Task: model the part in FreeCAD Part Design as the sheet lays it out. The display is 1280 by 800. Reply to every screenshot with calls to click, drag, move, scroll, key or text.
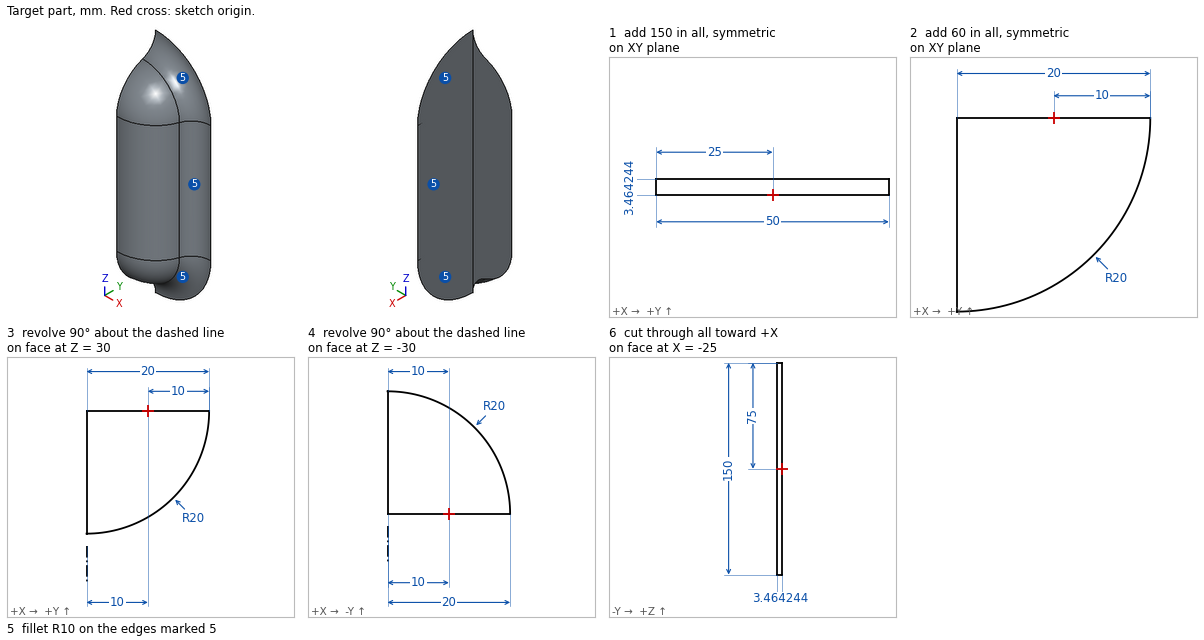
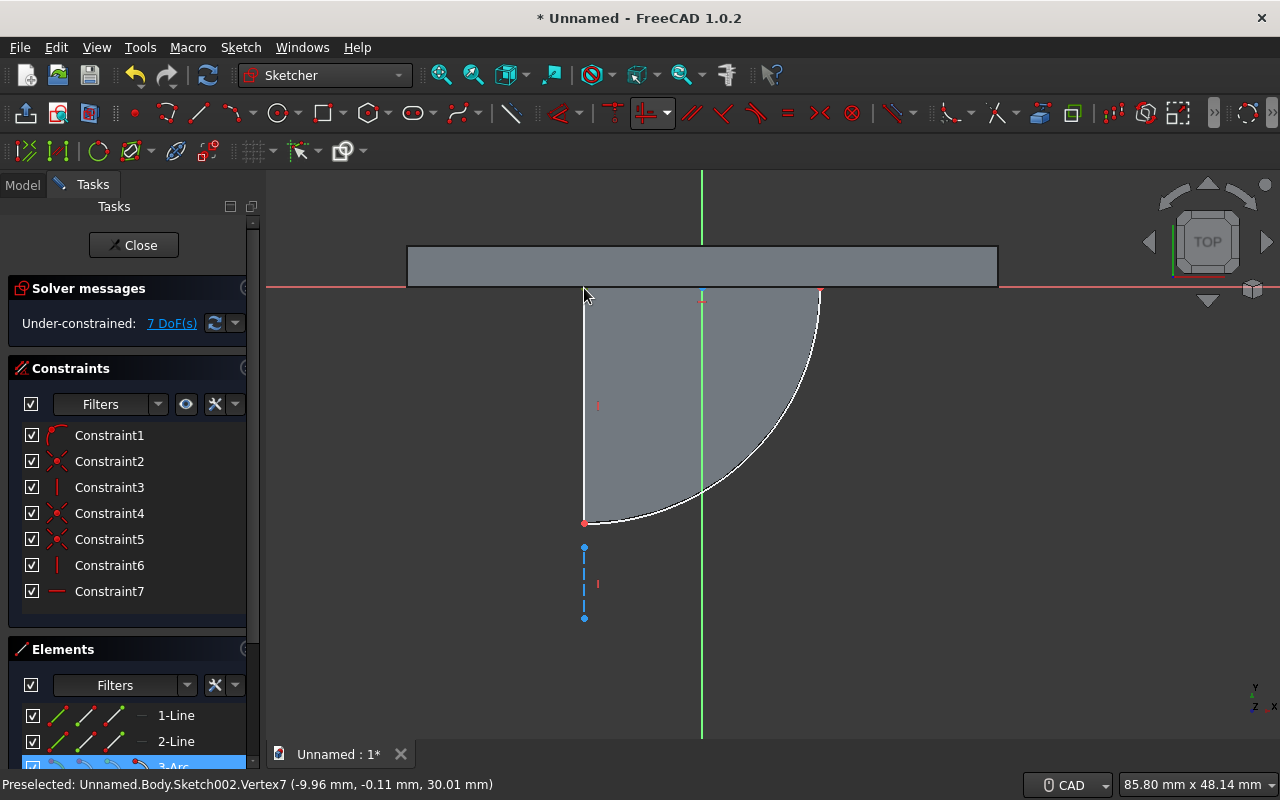
click(353, 287)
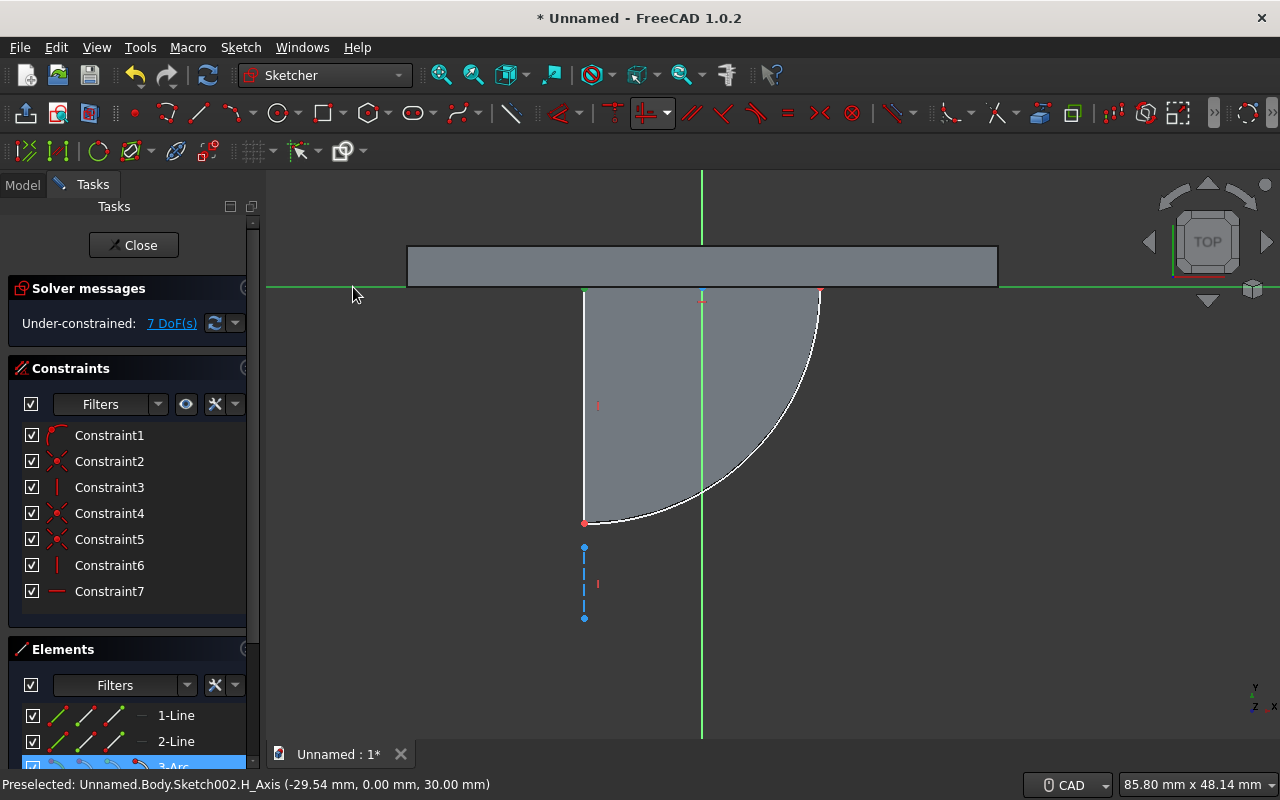
click(614, 114)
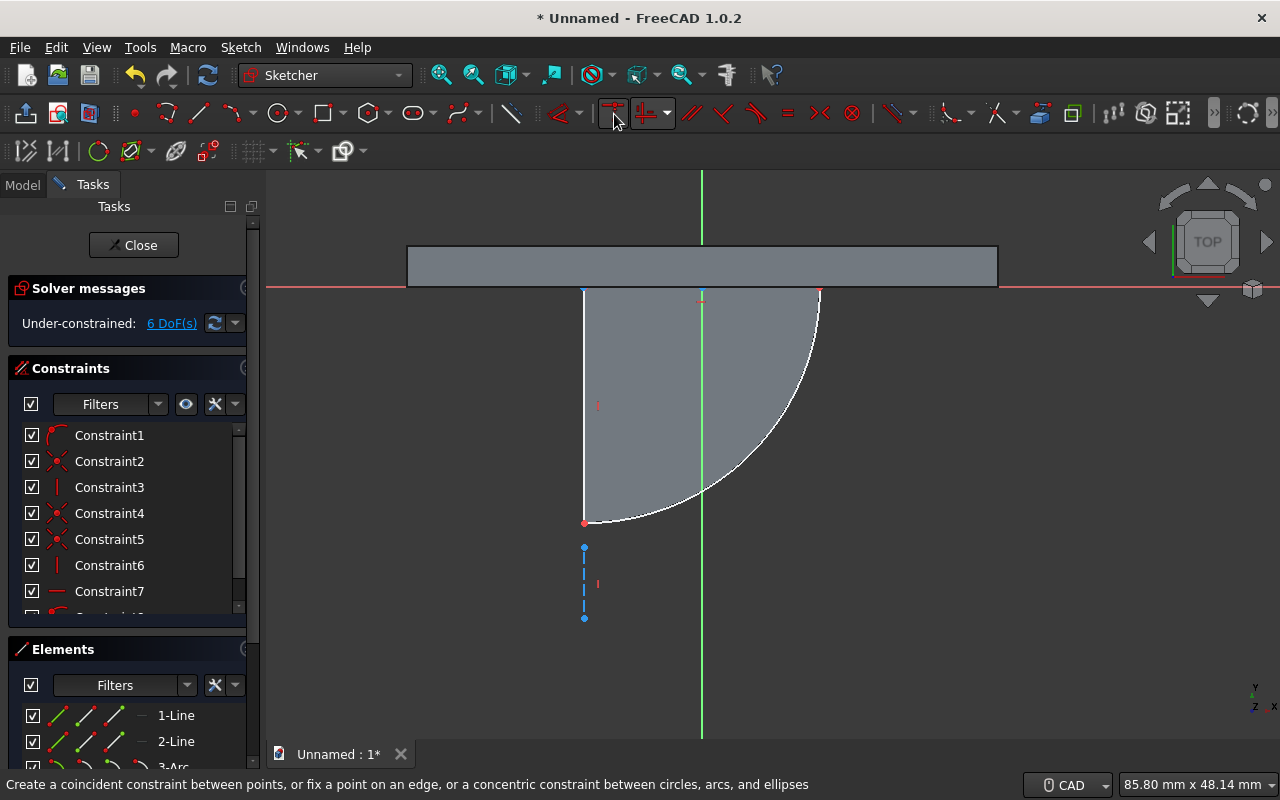
click(558, 114)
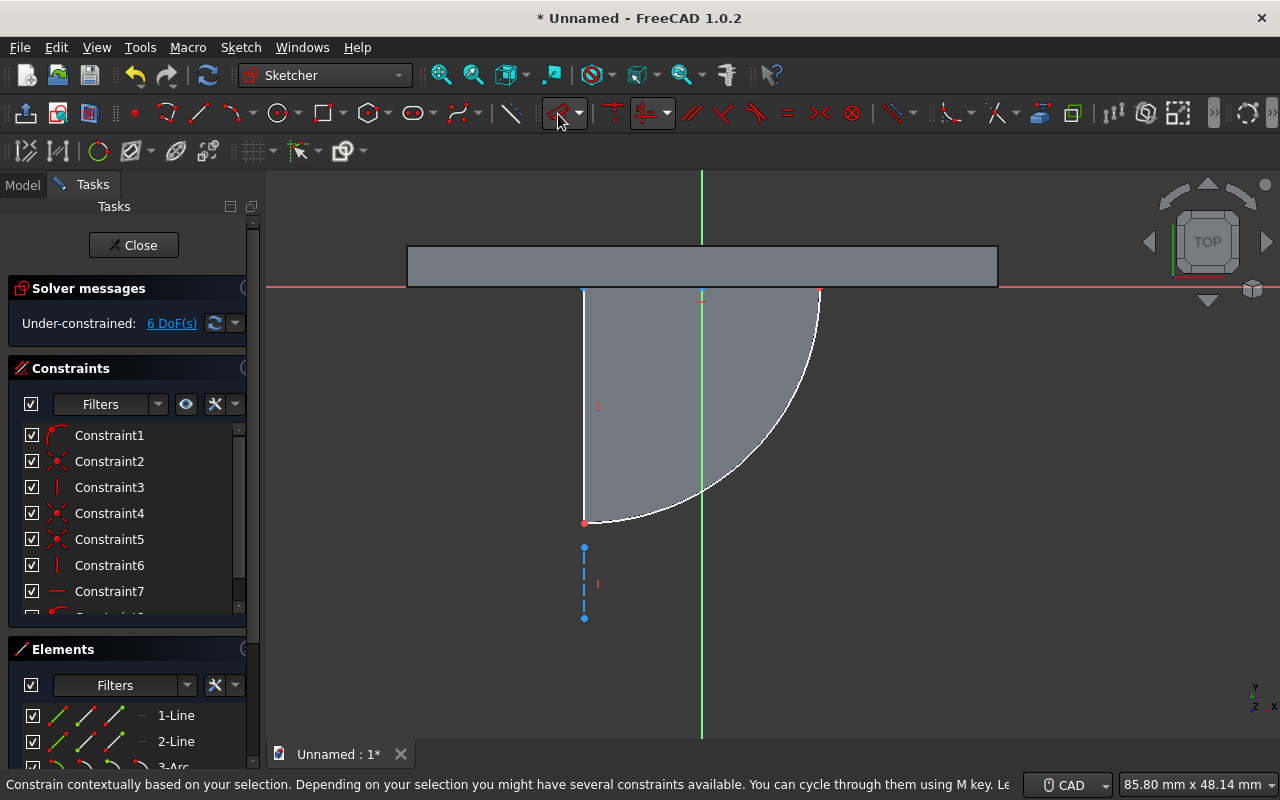
scroll(691, 497, up, 2)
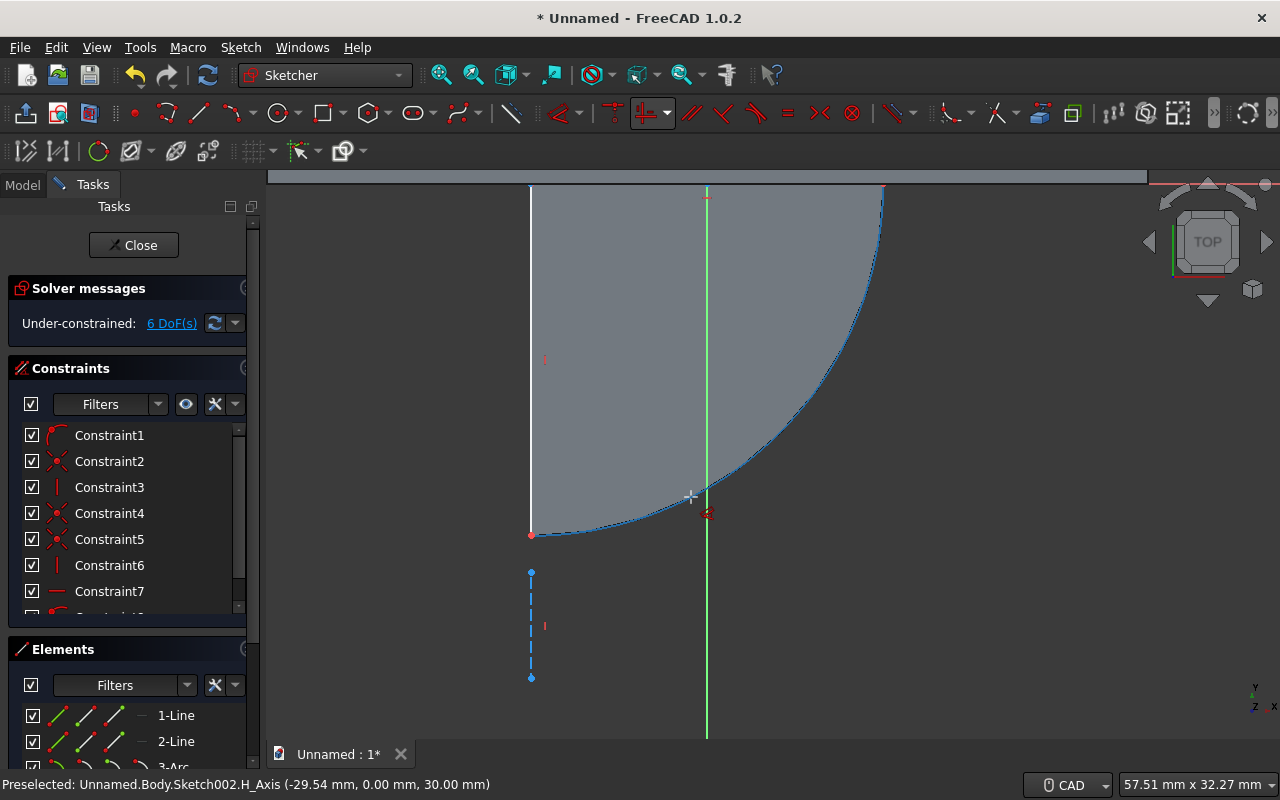
click(691, 497)
click(848, 400)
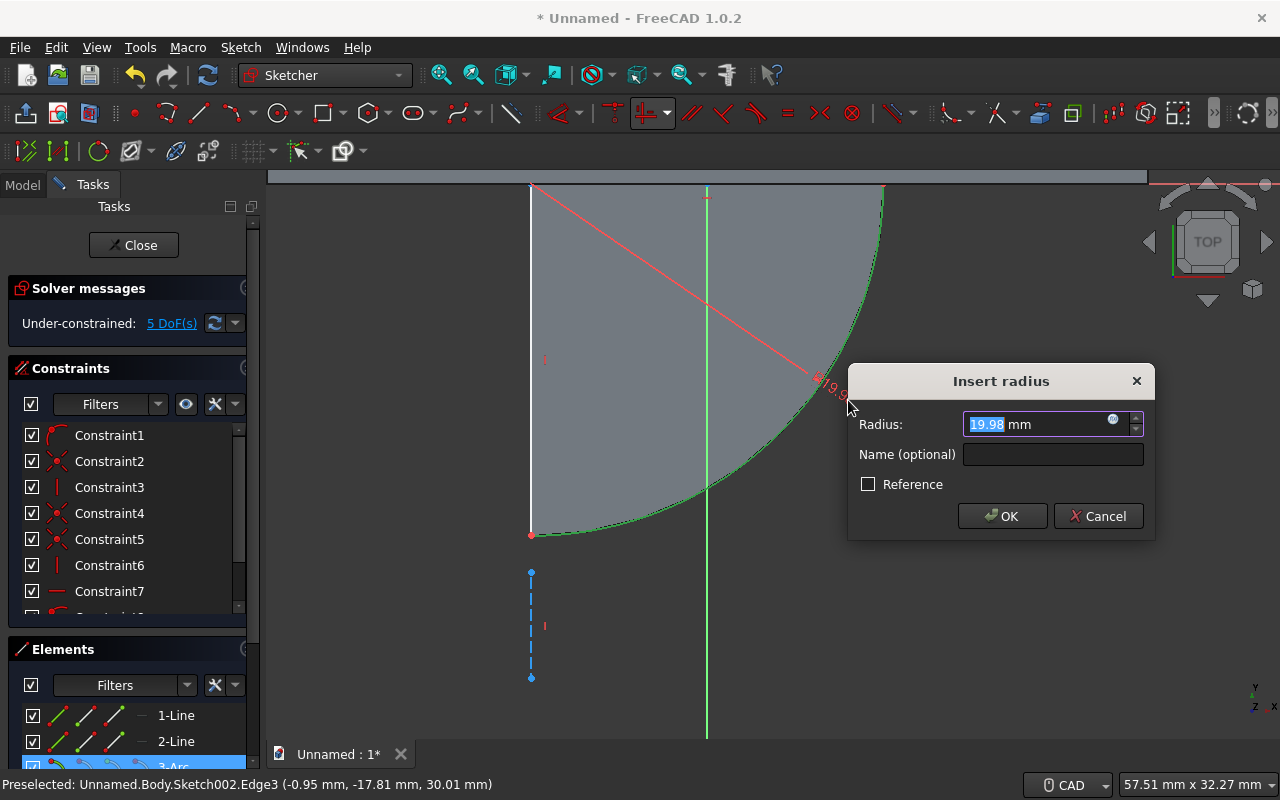
text(20)
key(Return)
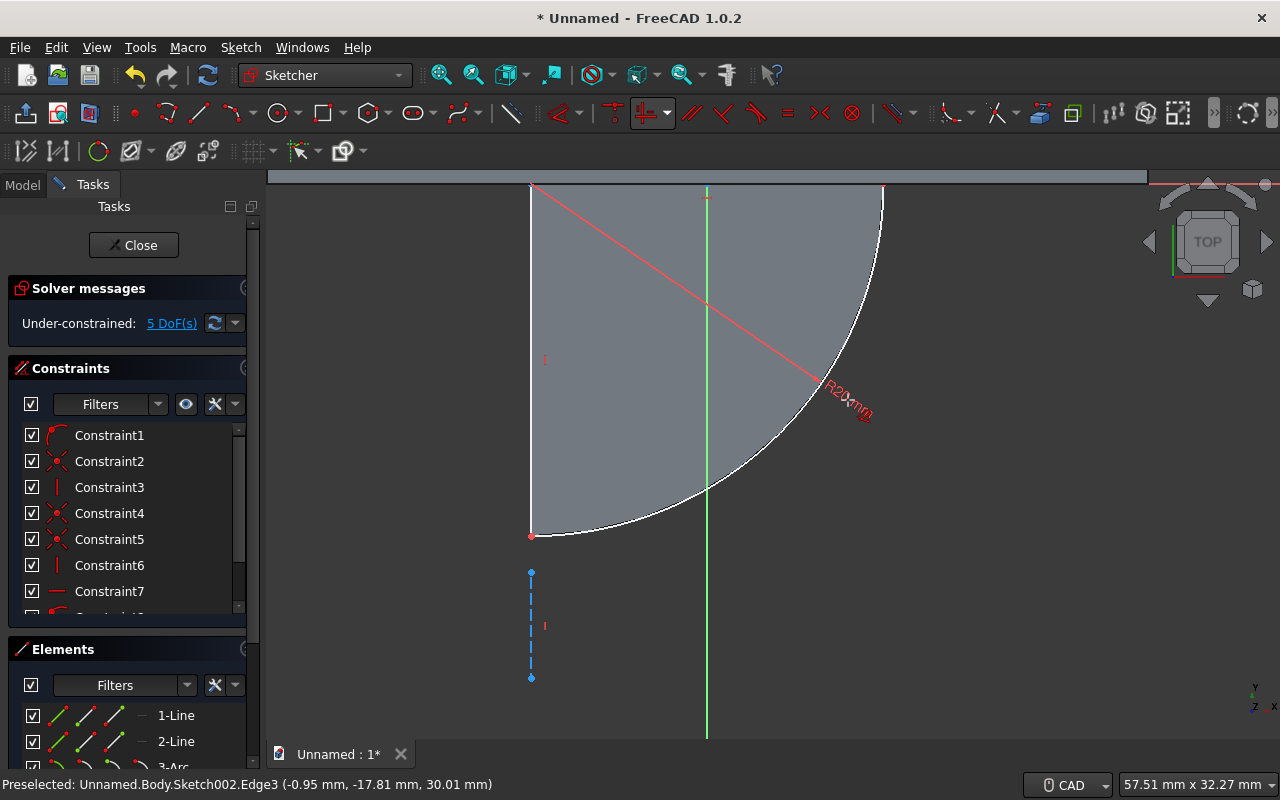
scroll(698, 504, down, 2)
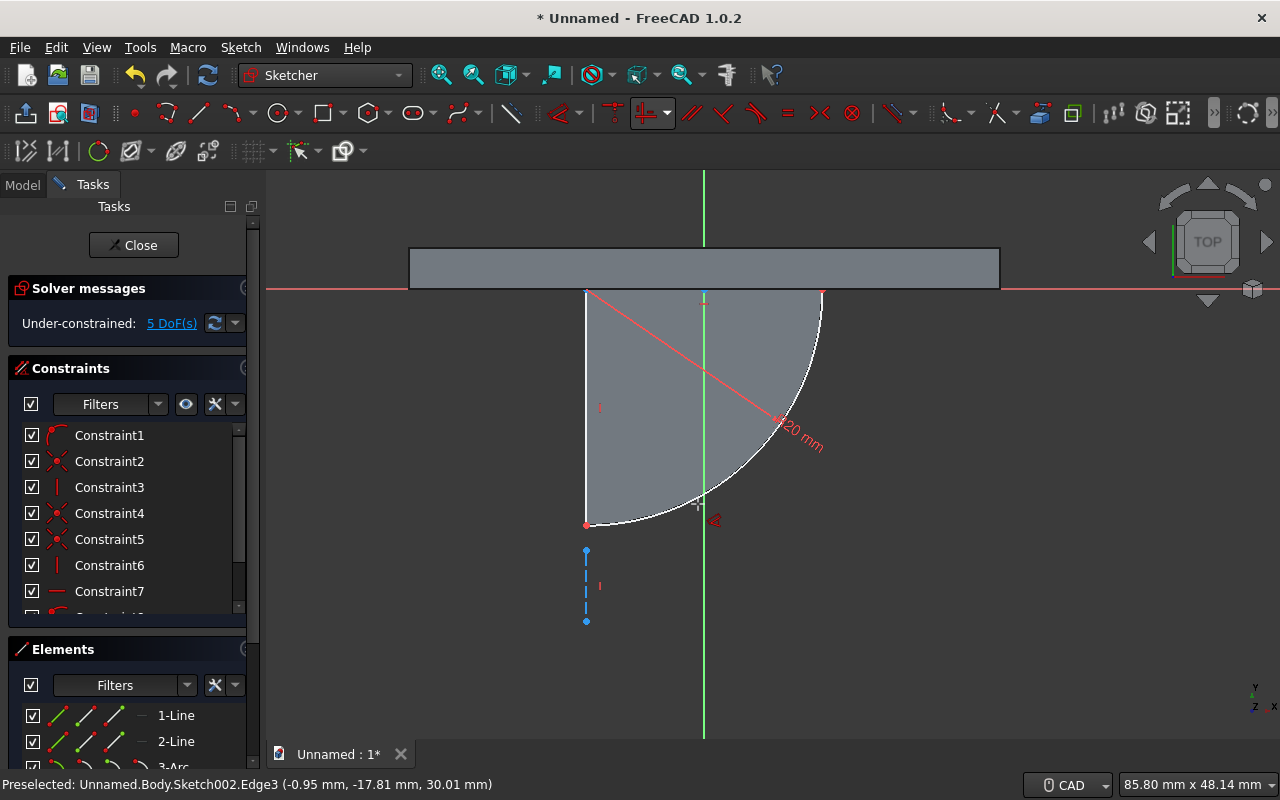
click(752, 289)
click(650, 255)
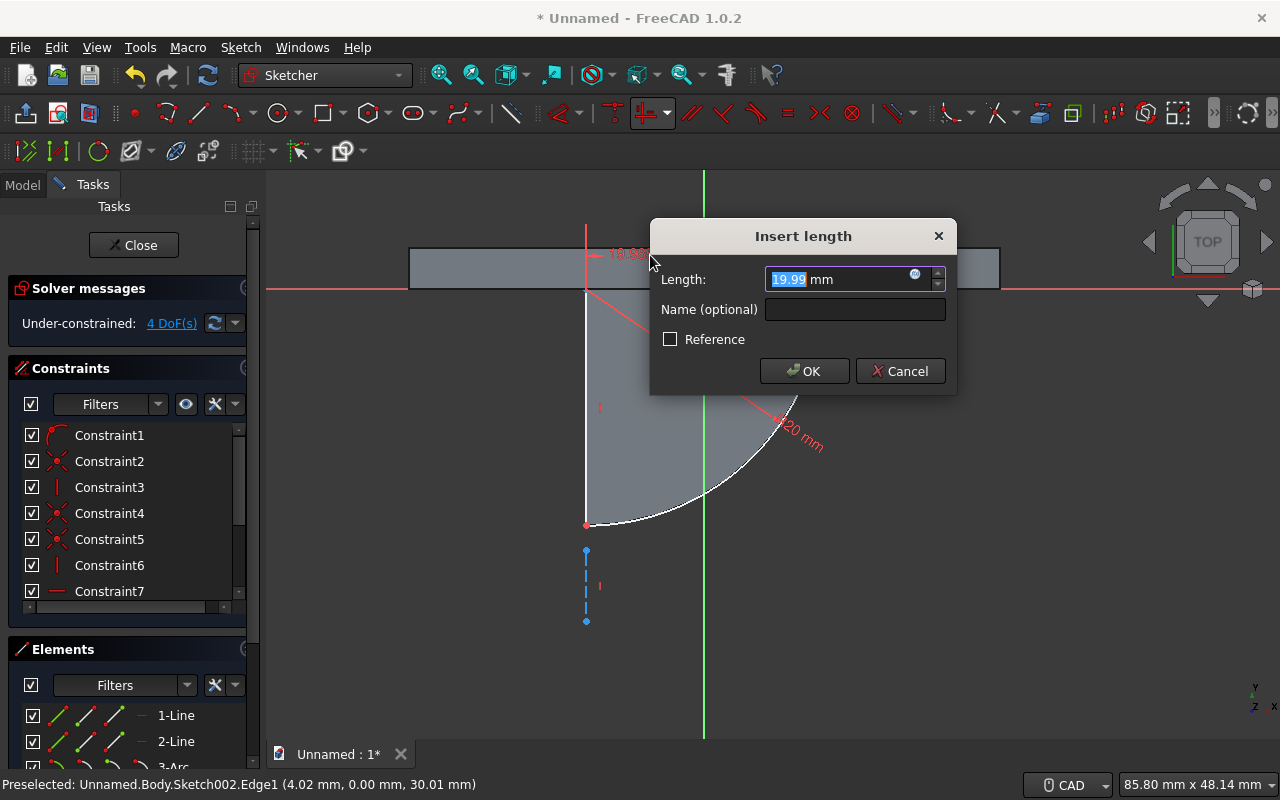
text(20)
key(Return)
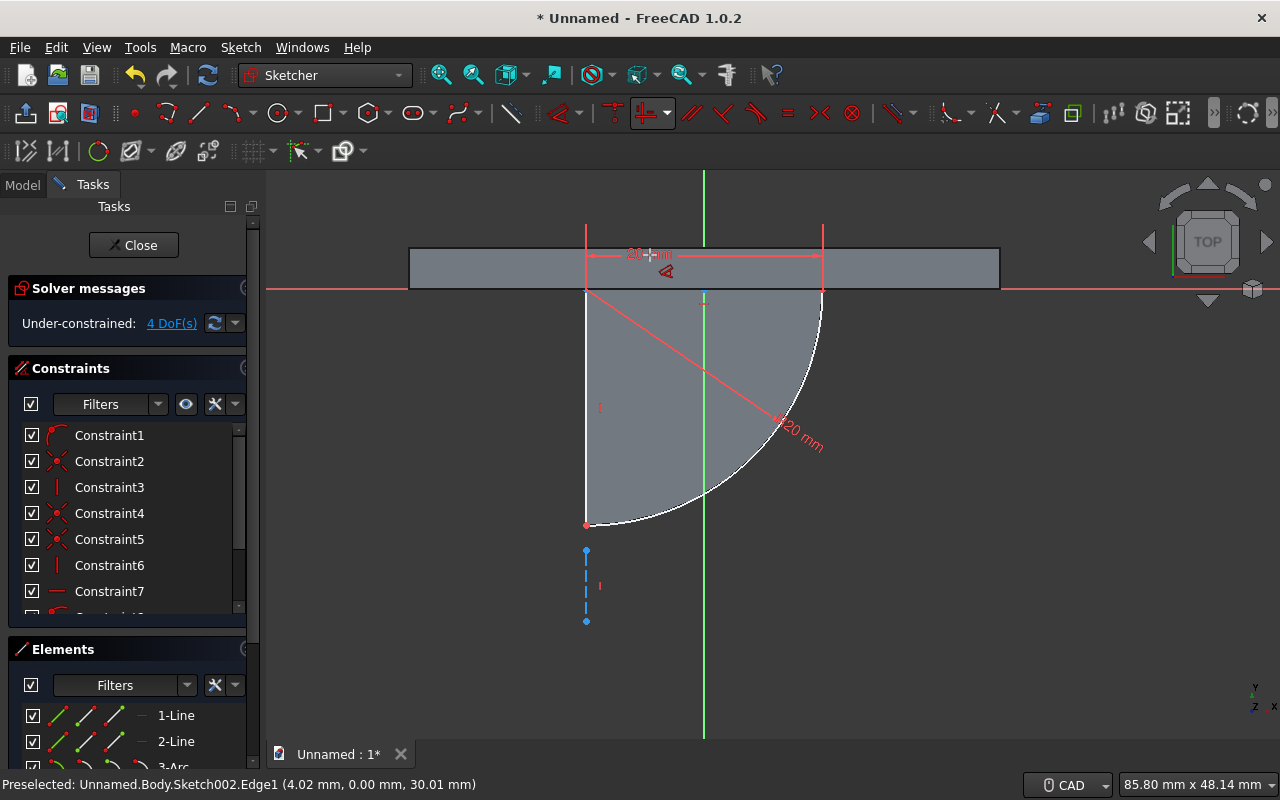
click(823, 289)
click(763, 255)